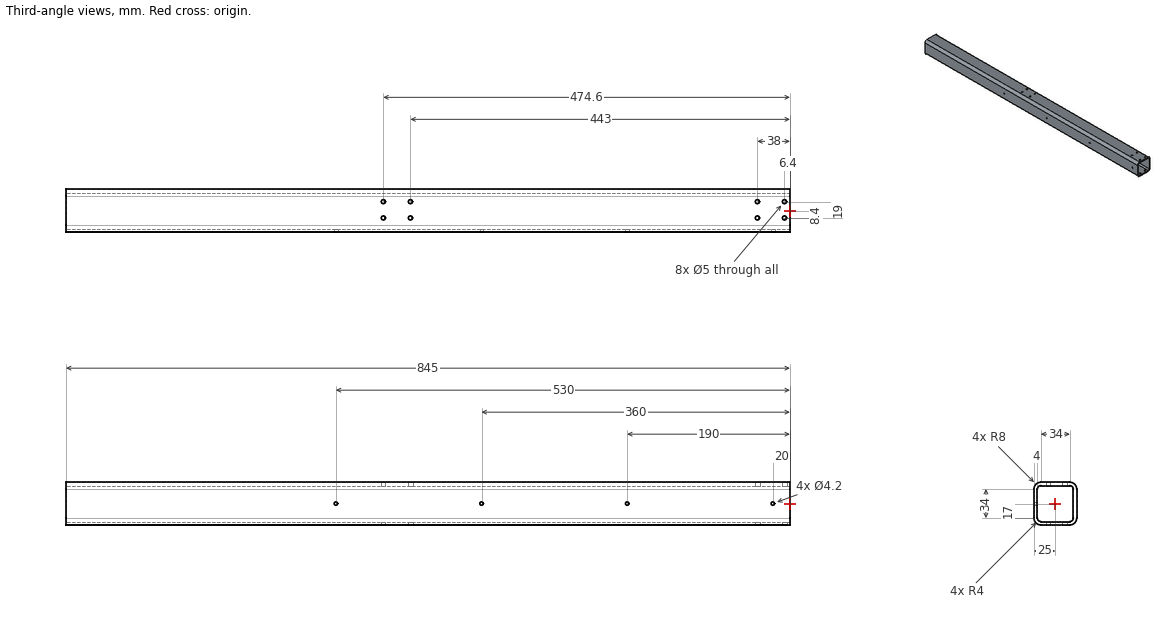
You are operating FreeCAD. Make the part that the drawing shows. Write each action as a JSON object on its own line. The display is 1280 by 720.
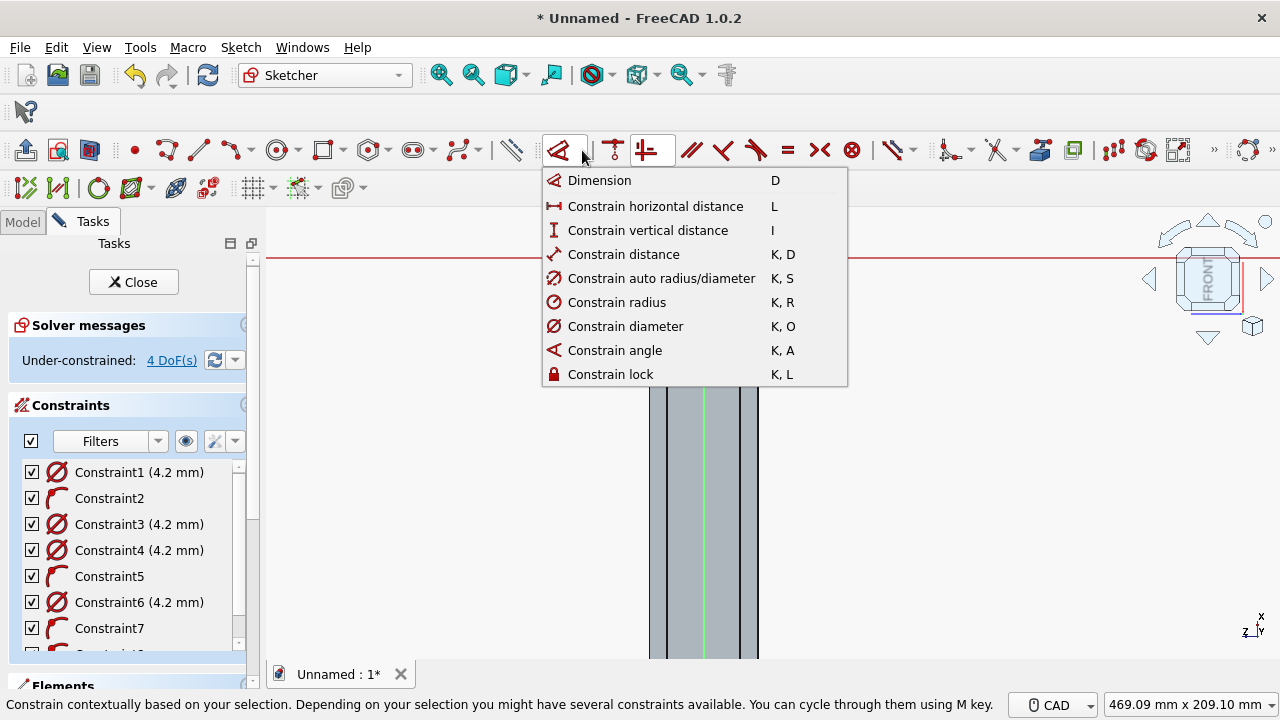
{"action": "left_click", "coordinate": [695, 230]}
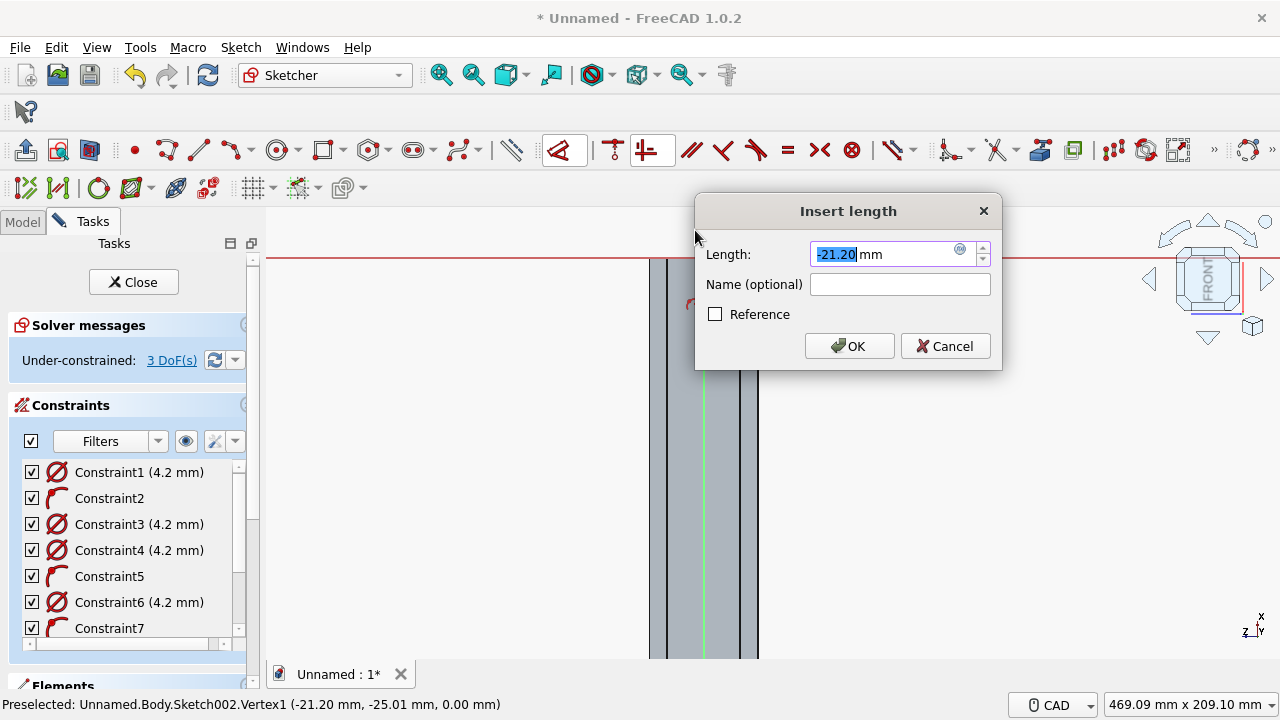
{"action": "type", "text": "-20"}
{"action": "key", "text": "Return"}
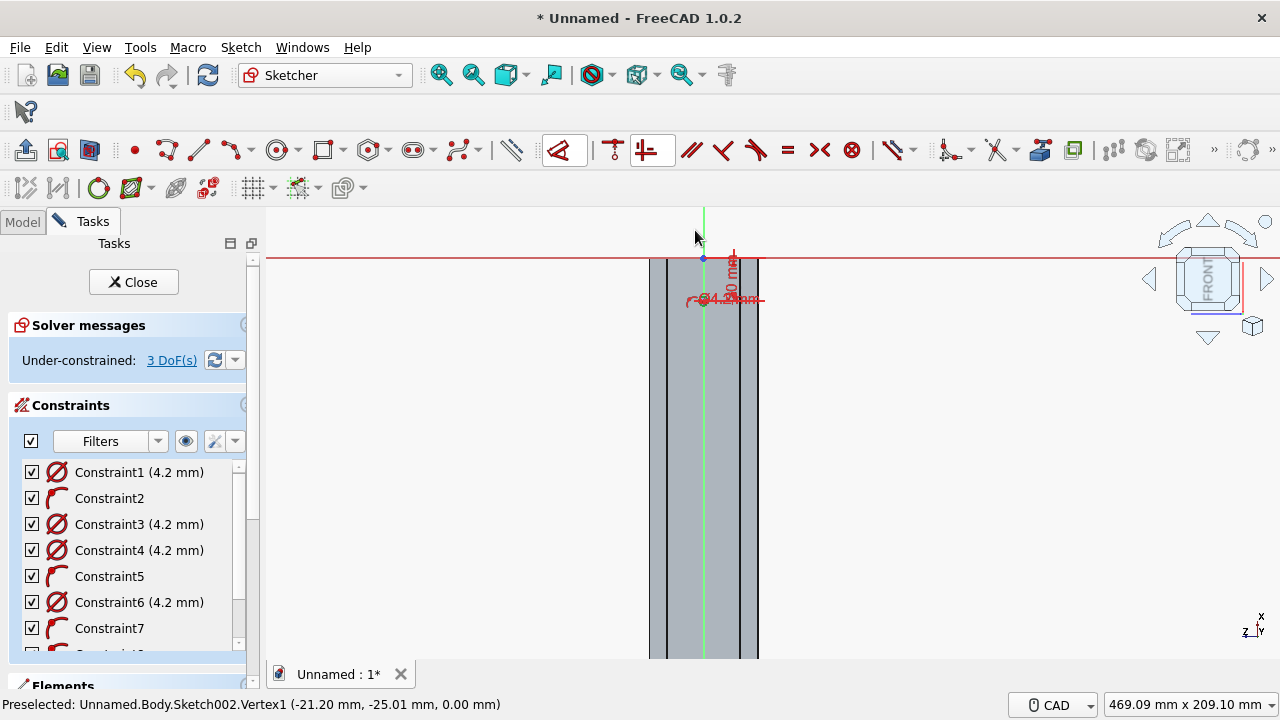
{"action": "scroll", "coordinate": [705, 302], "scroll_direction": "down", "scroll_amount": 7}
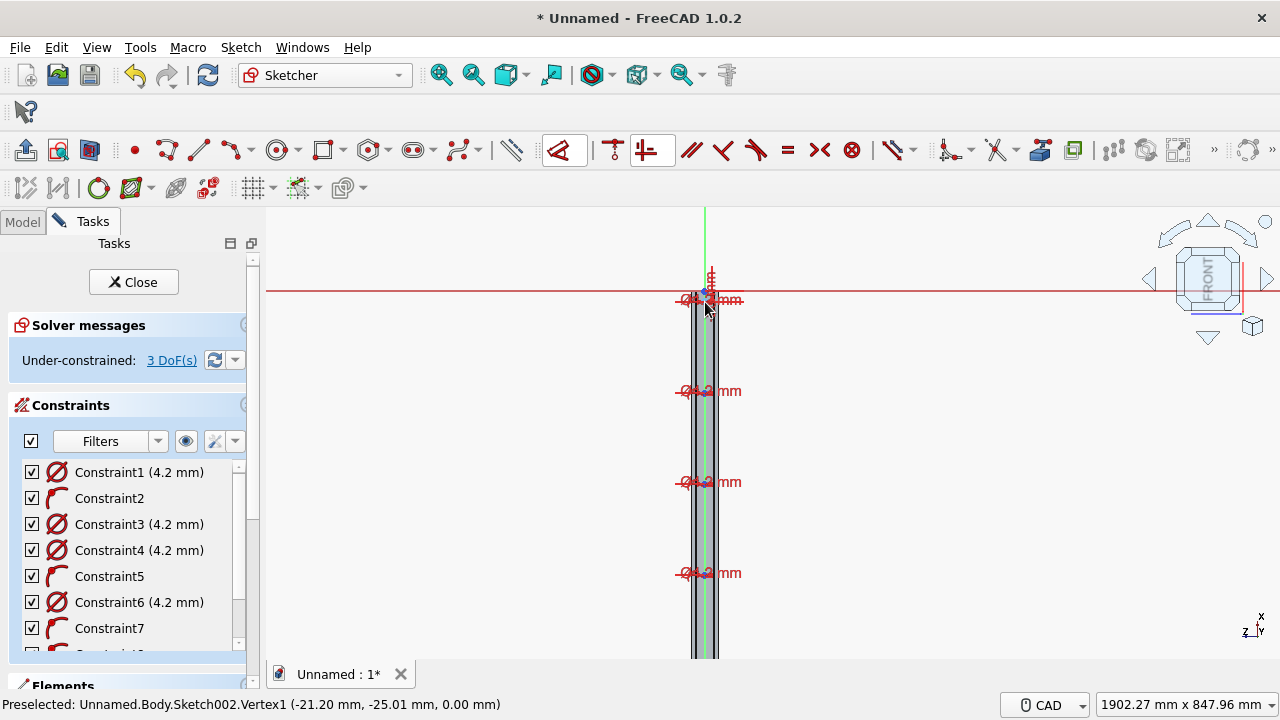
{"action": "left_click", "coordinate": [705, 393]}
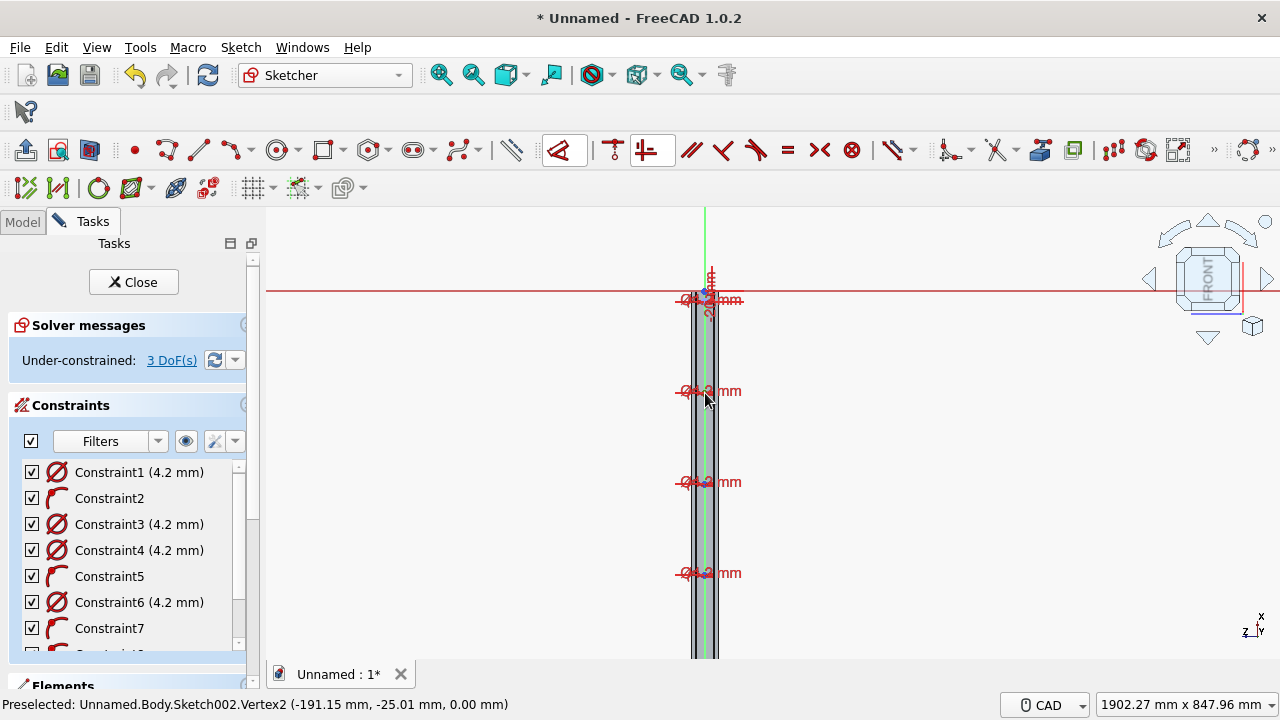
{"action": "key", "text": "i"}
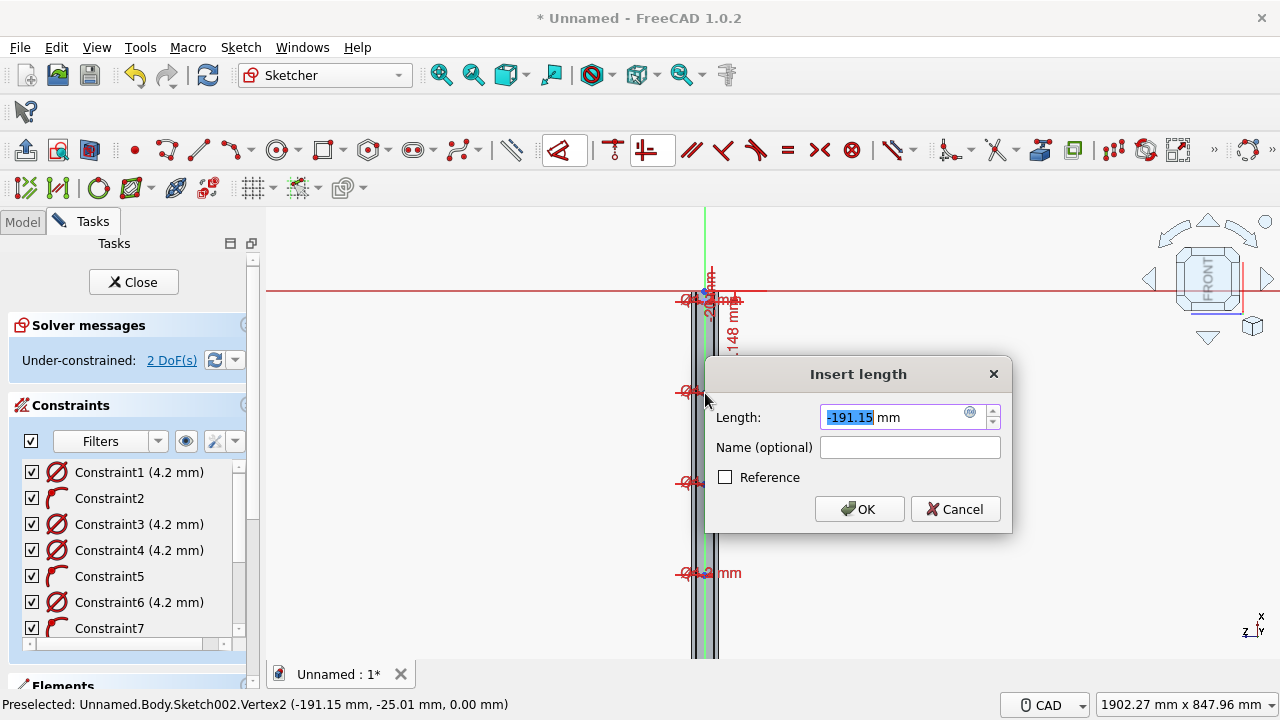
{"action": "type", "text": "-190"}
{"action": "key", "text": "Return"}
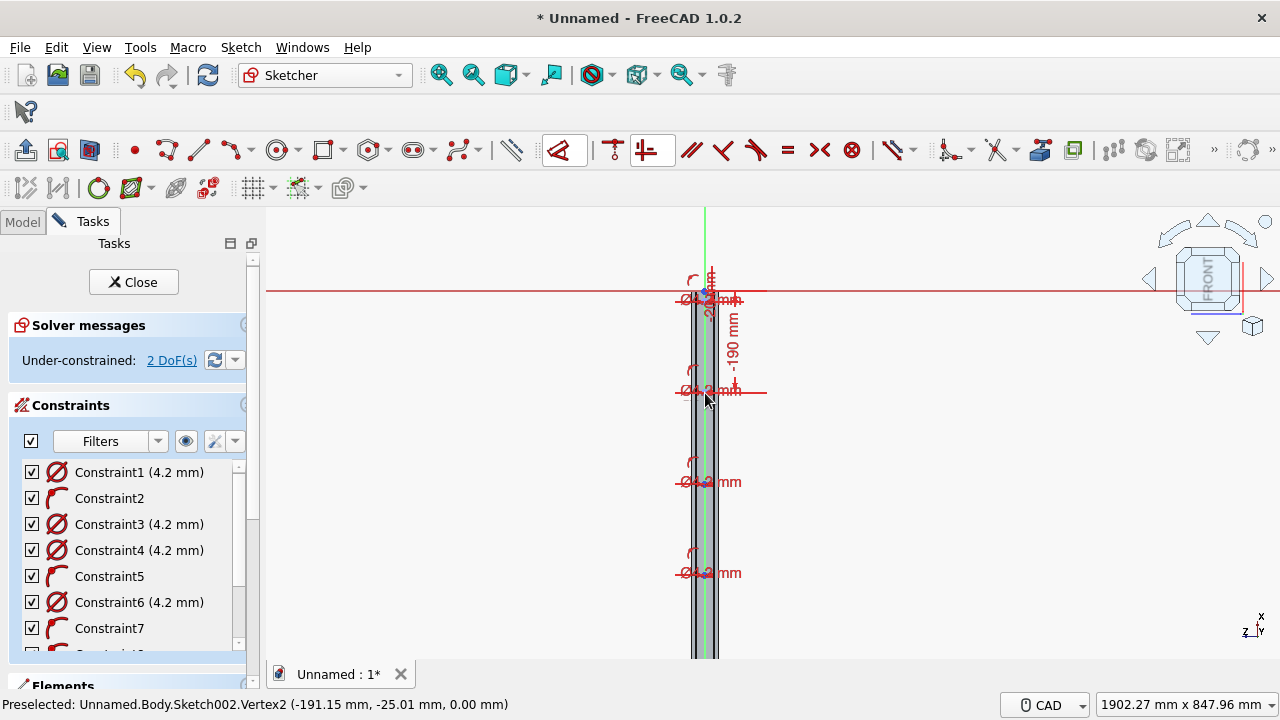
{"action": "left_click", "coordinate": [705, 484]}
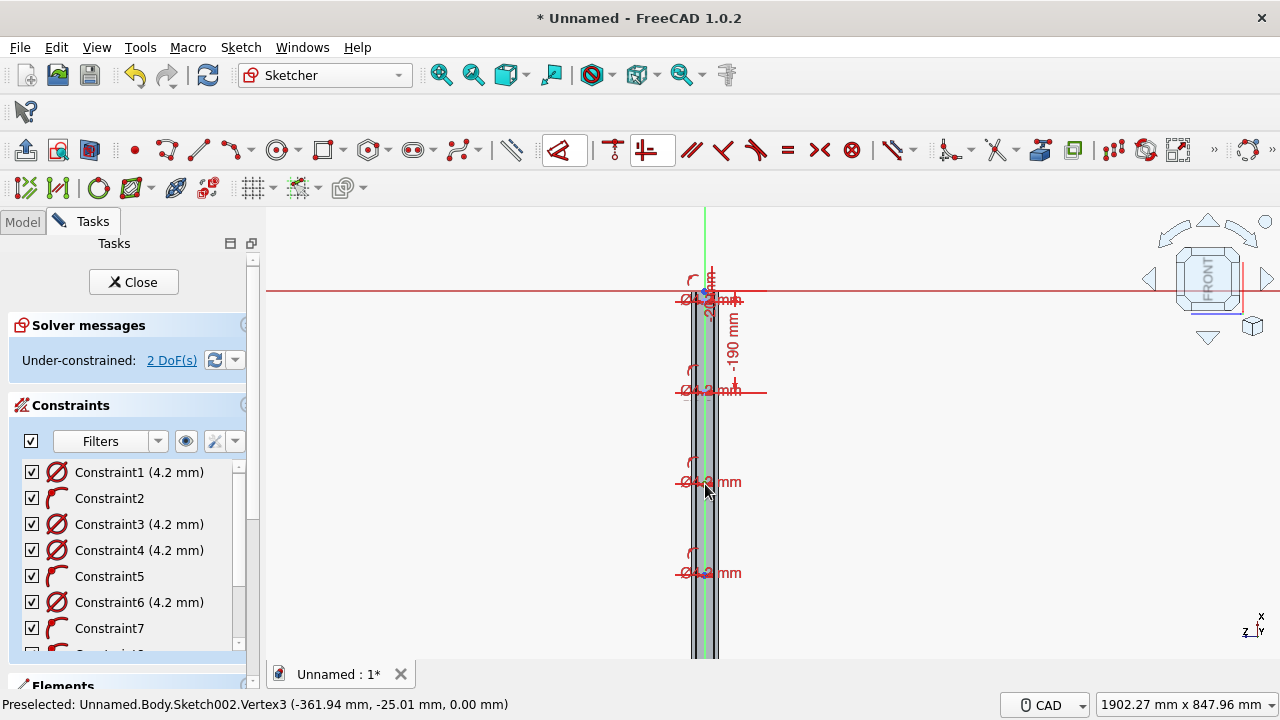
{"action": "left_click", "coordinate": [582, 150]}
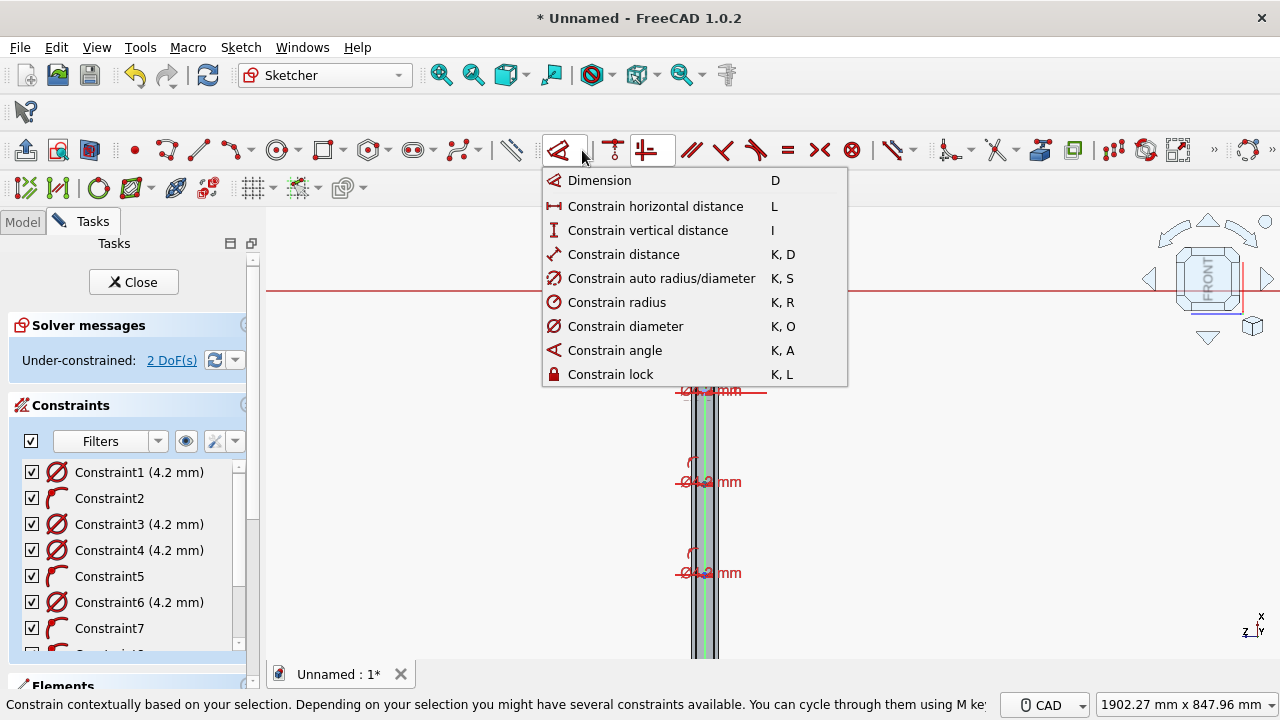
{"action": "left_click", "coordinate": [695, 230]}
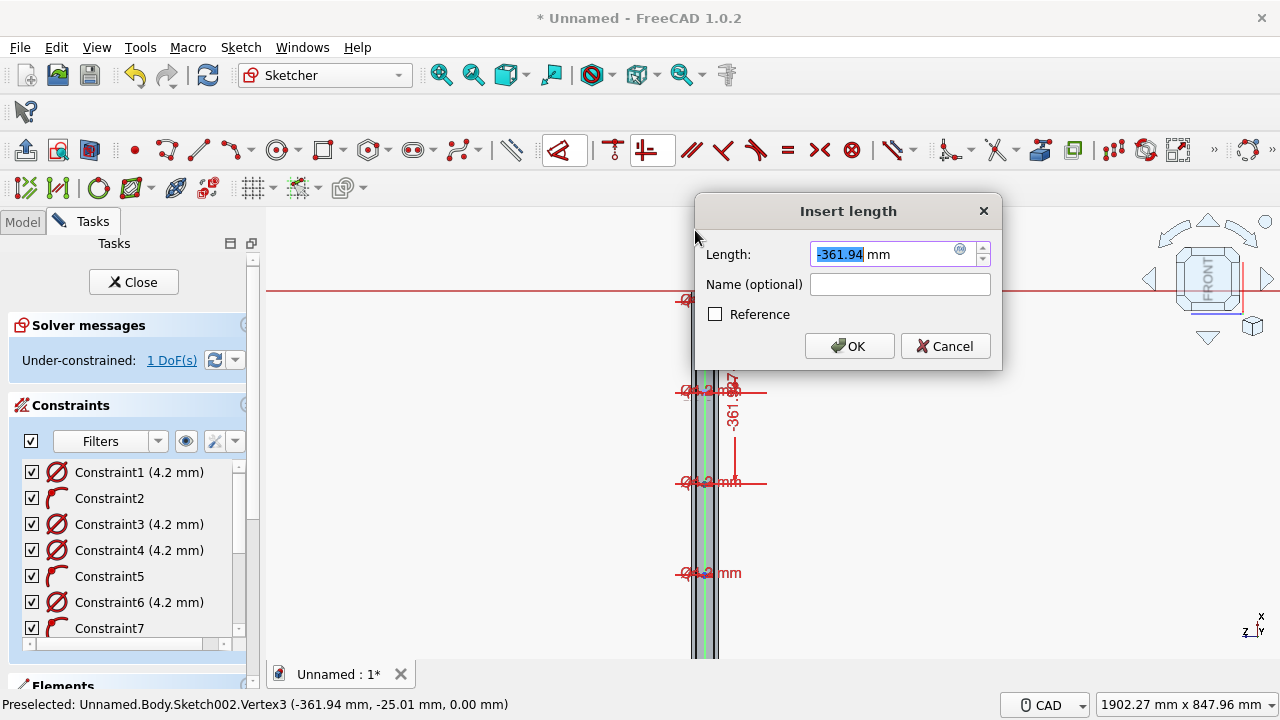
{"action": "type", "text": "-360"}
{"action": "key", "text": "Return"}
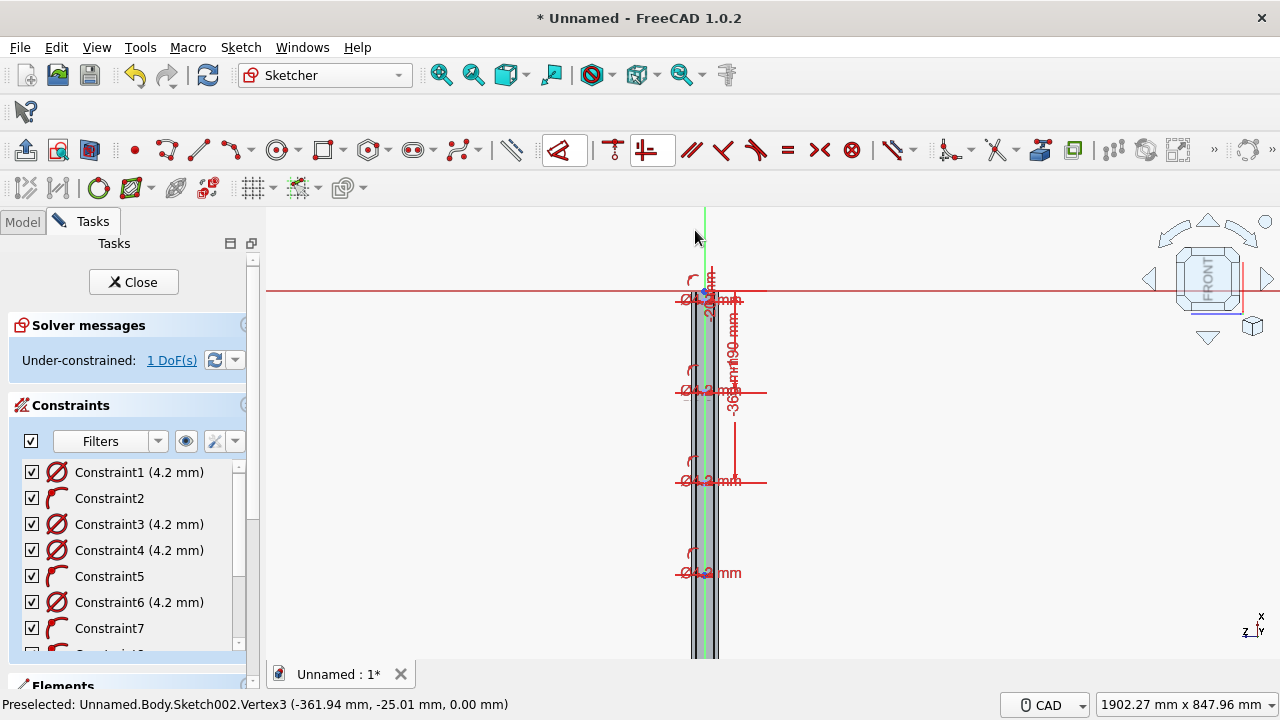
{"action": "left_click", "coordinate": [705, 575]}